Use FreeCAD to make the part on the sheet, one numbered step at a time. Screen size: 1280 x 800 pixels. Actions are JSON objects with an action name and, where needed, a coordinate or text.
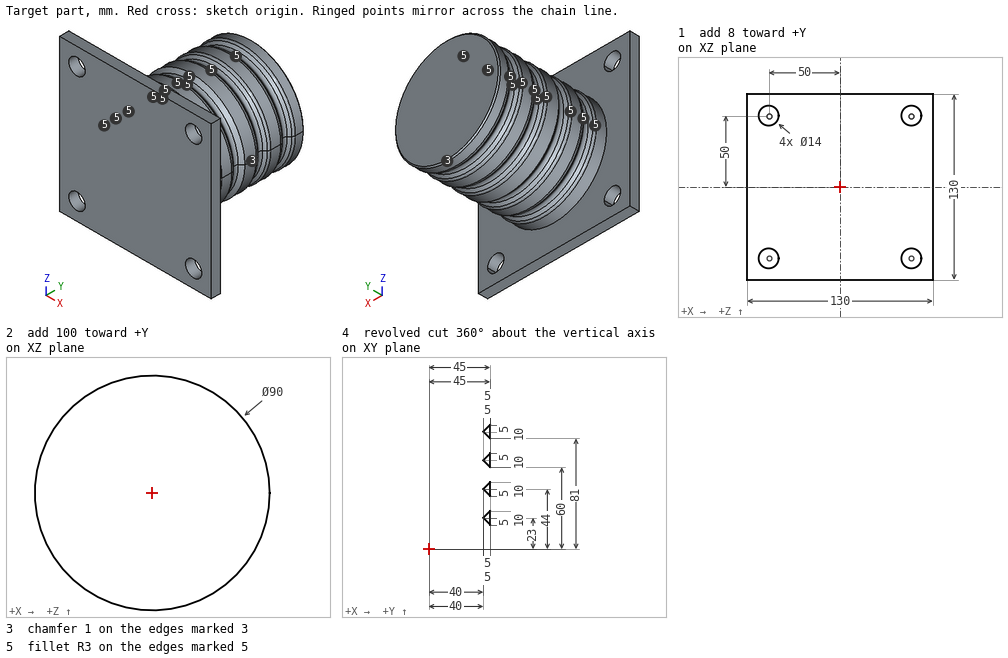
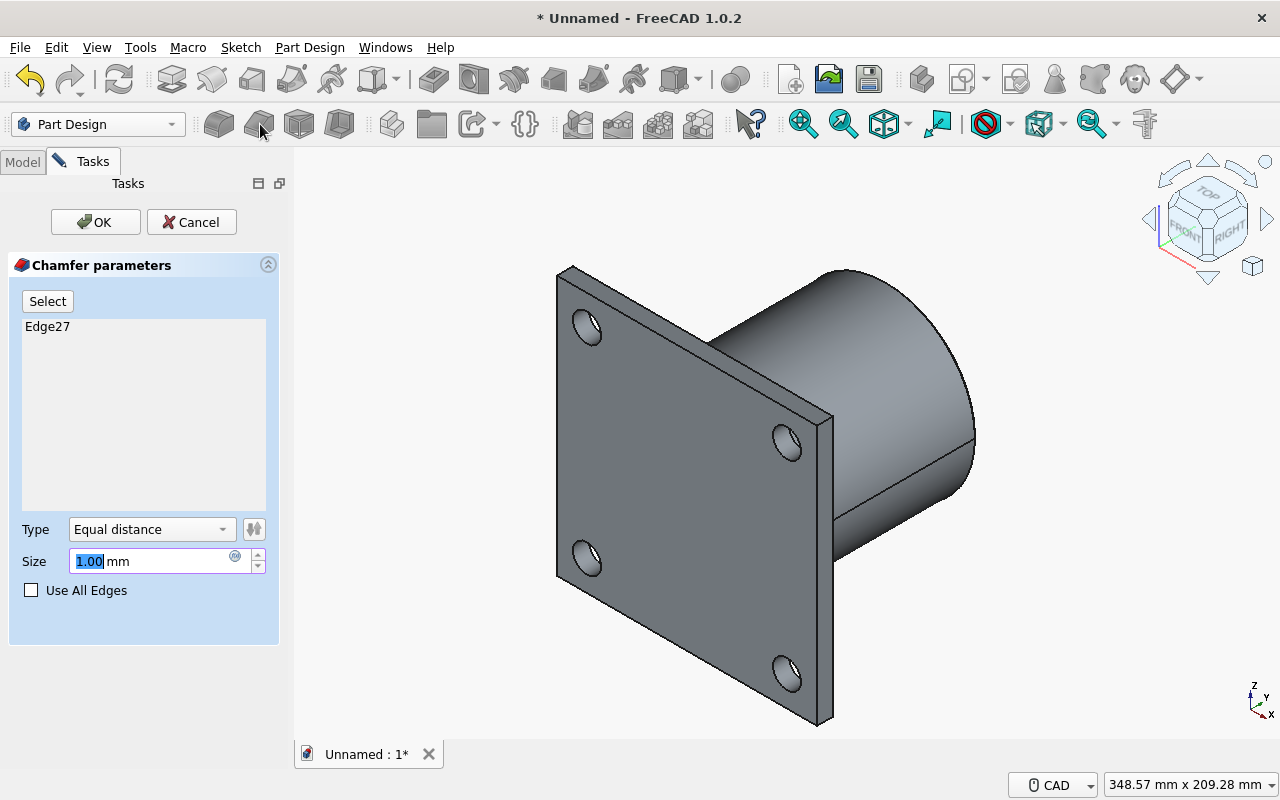
{"action": "type", "text": "1"}
{"action": "key", "text": "Tab"}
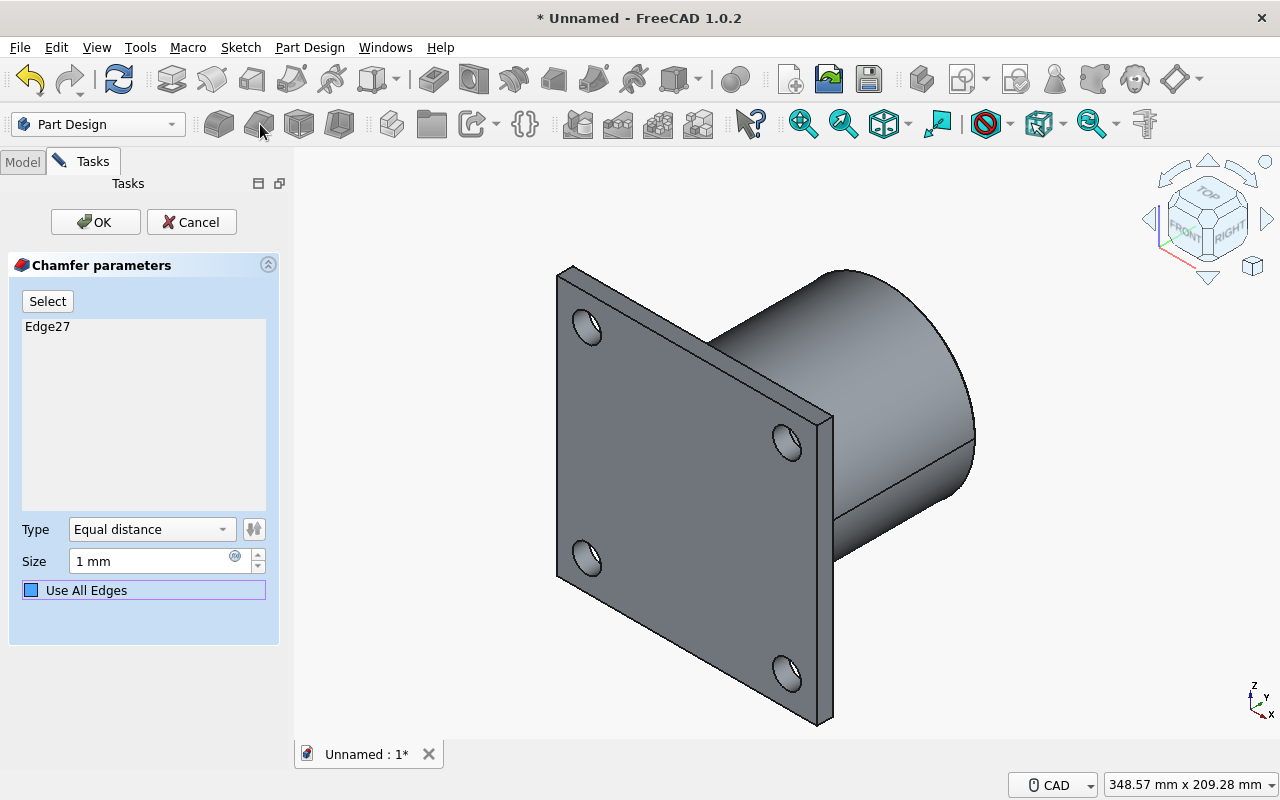
{"action": "left_click", "coordinate": [96, 222]}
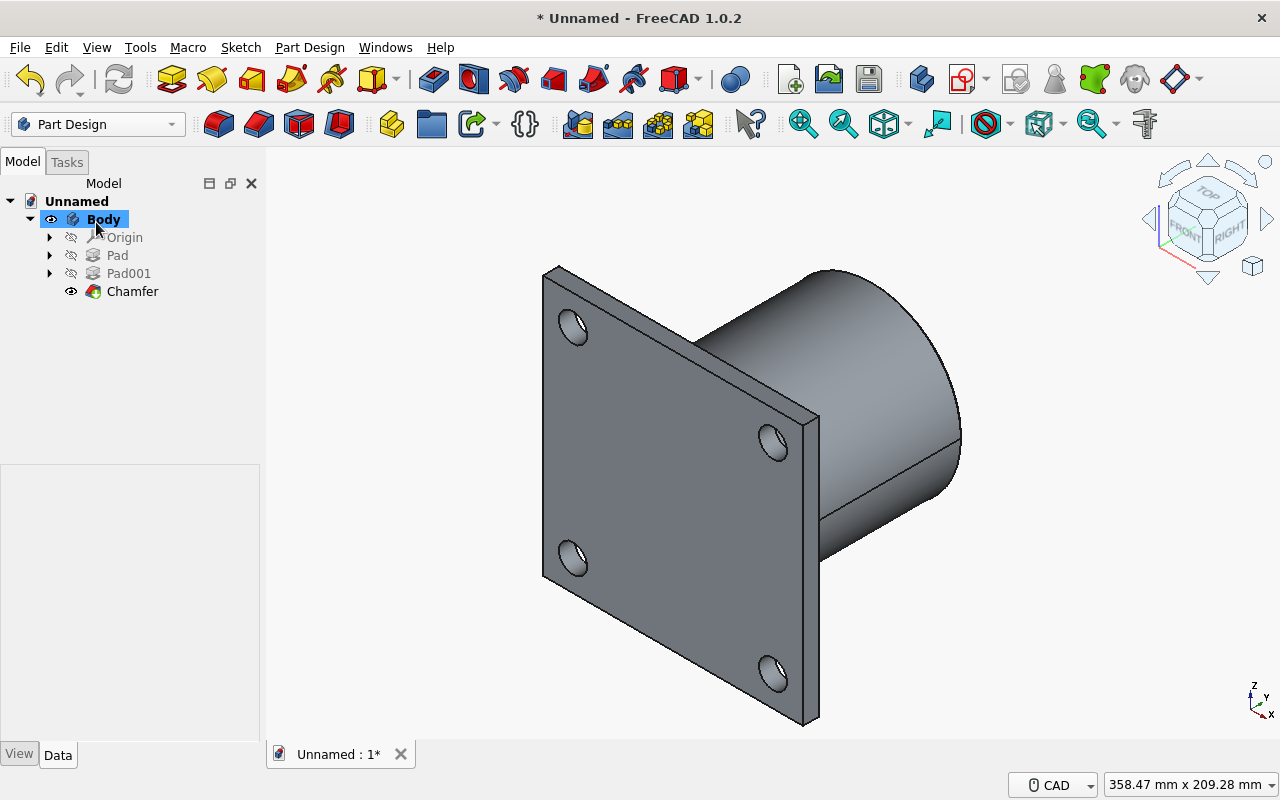
{"action": "left_click", "coordinate": [962, 80]}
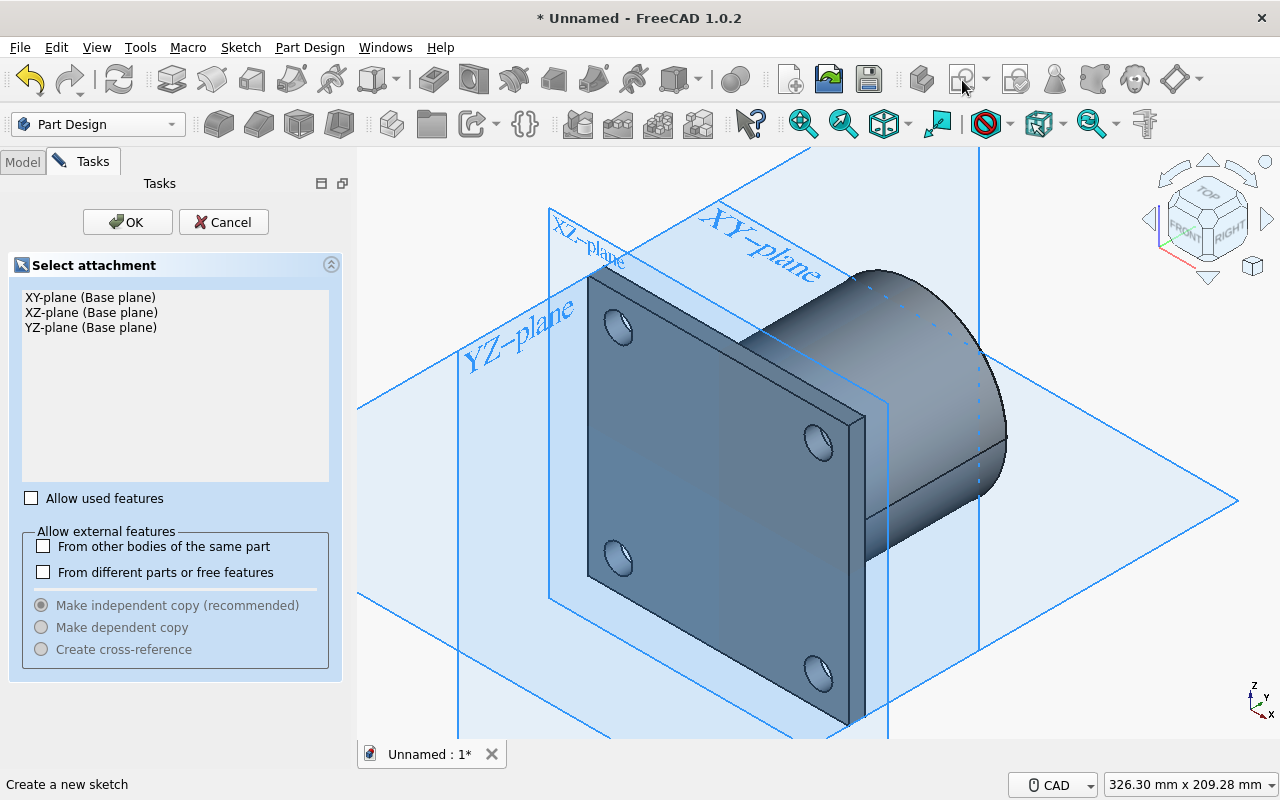
{"action": "left_click", "coordinate": [82, 298]}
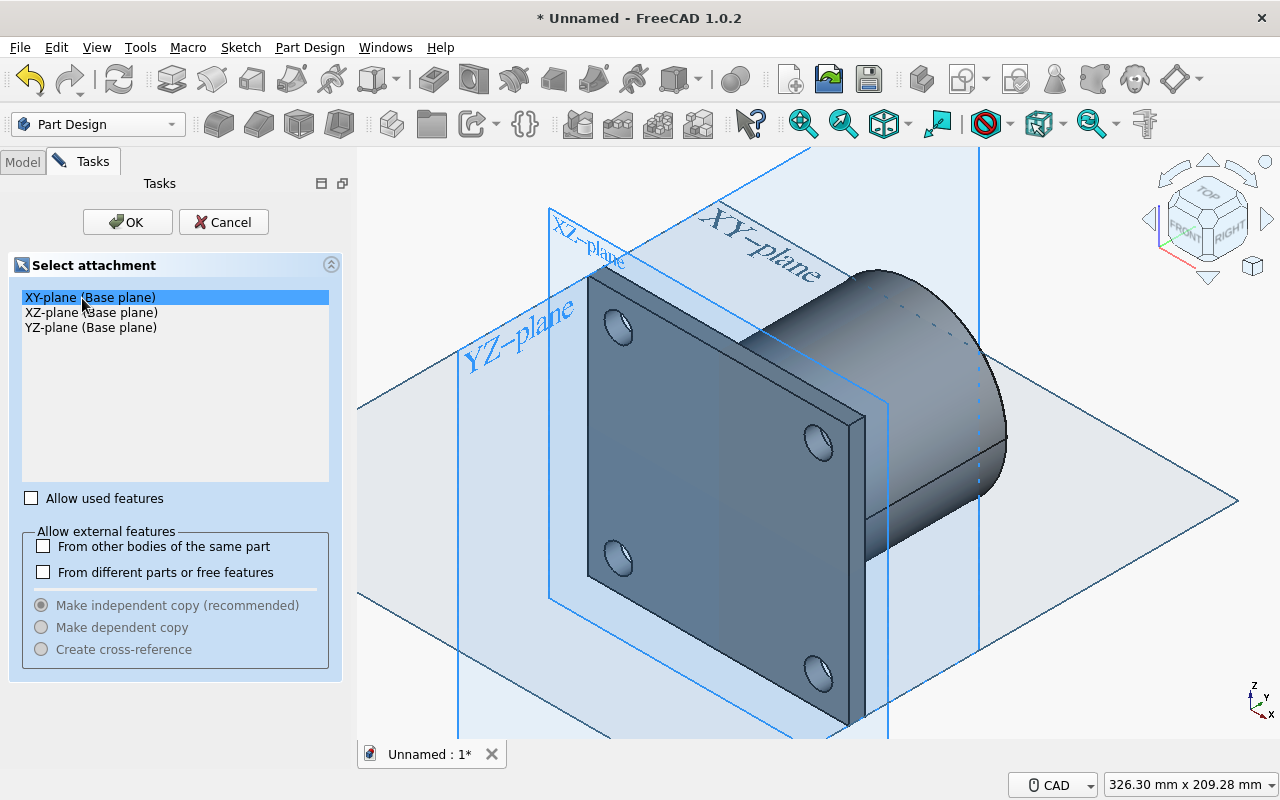
{"action": "left_click", "coordinate": [128, 222]}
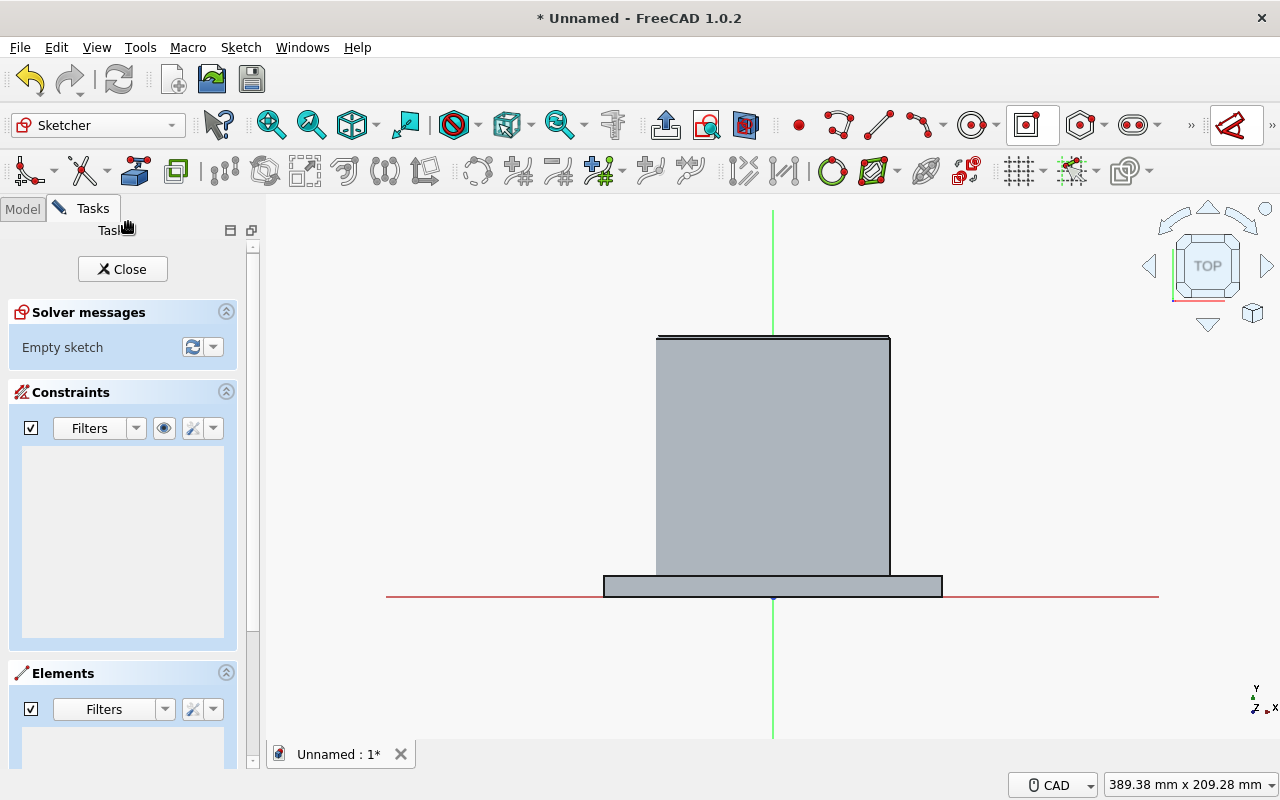
{"action": "left_click", "coordinate": [746, 126]}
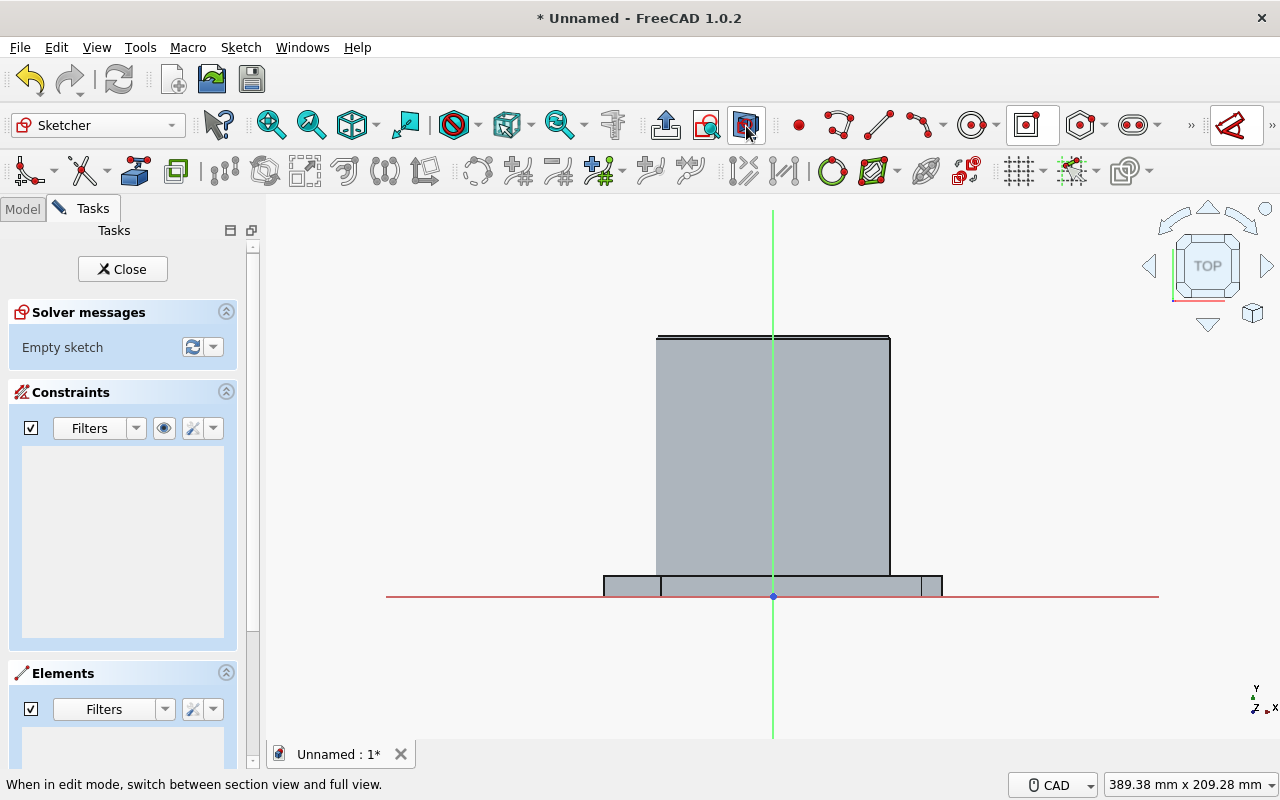
{"action": "scroll", "coordinate": [1090, 502], "scroll_direction": "up", "scroll_amount": 2}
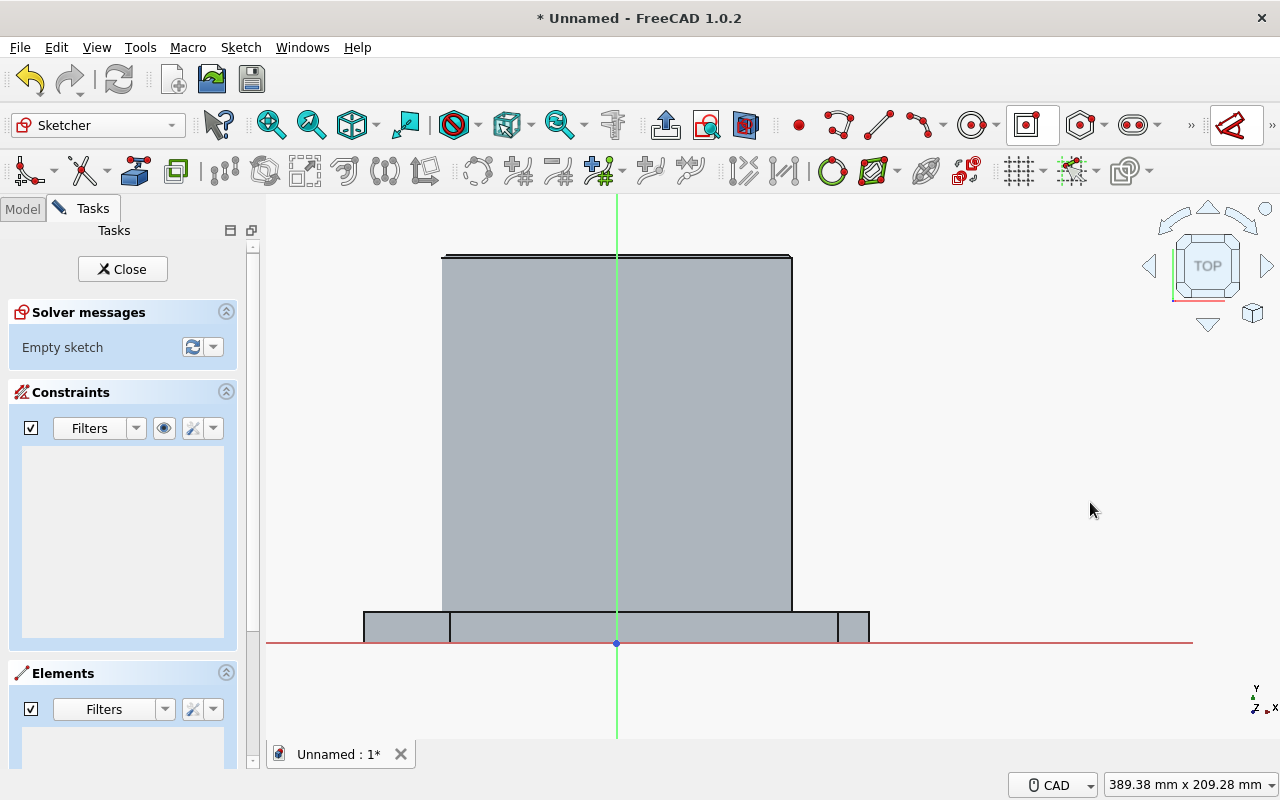
{"action": "left_click", "coordinate": [840, 126]}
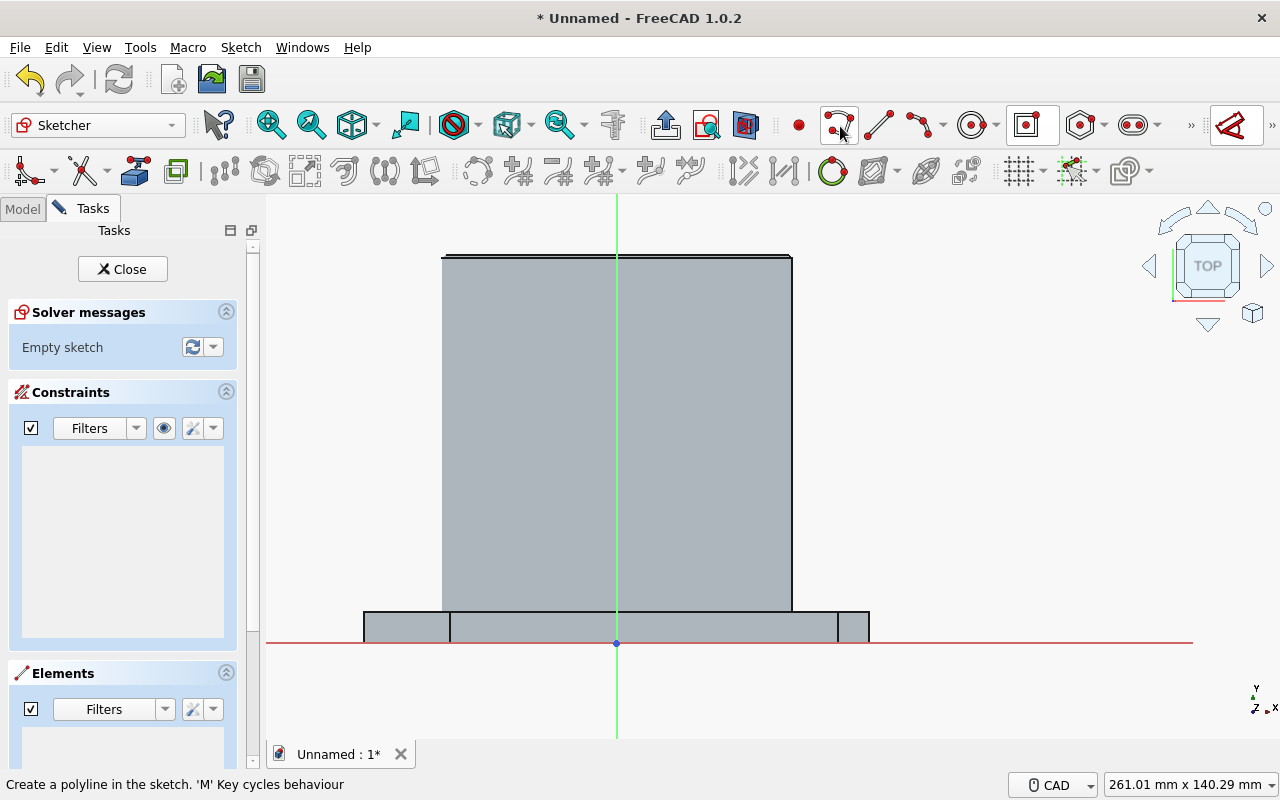
{"action": "left_click", "coordinate": [772, 554]}
{"action": "left_click", "coordinate": [792, 573]}
{"action": "left_click", "coordinate": [792, 534]}
{"action": "left_click", "coordinate": [772, 555]}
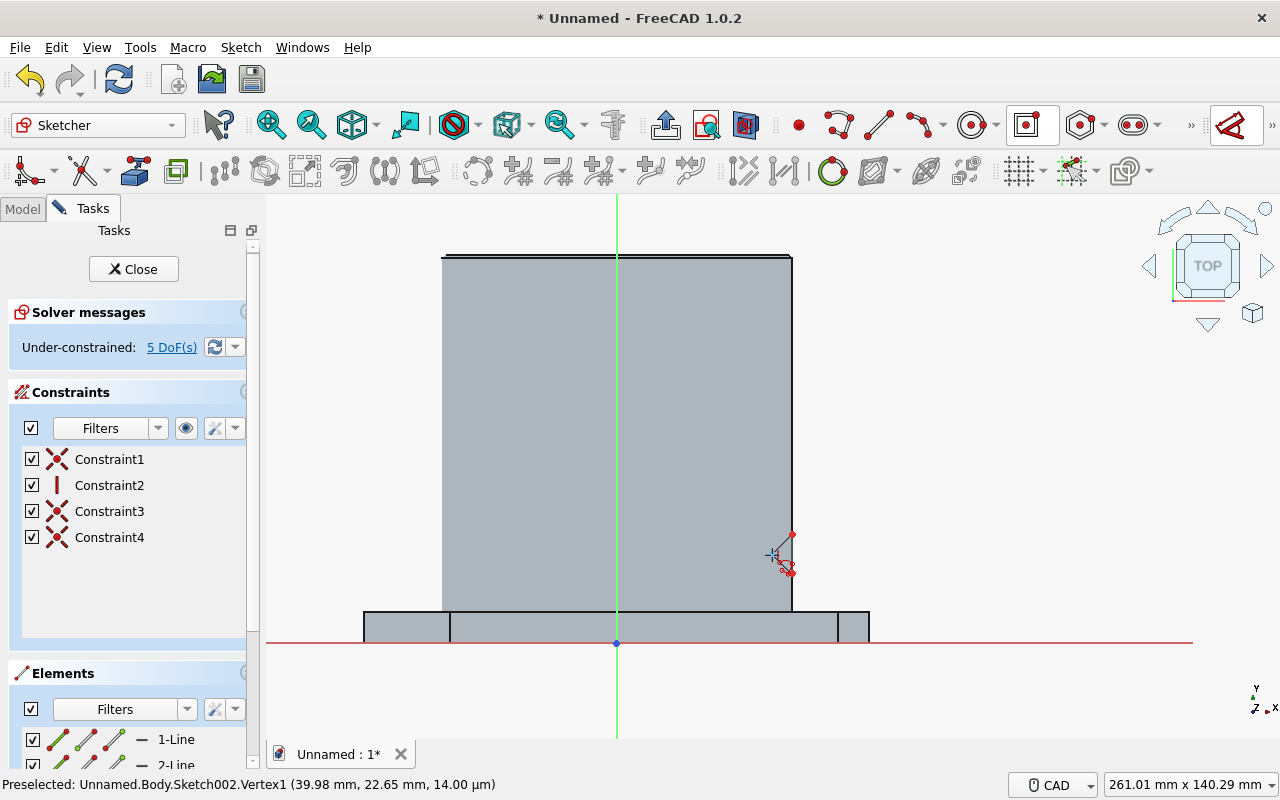
{"action": "left_click", "coordinate": [772, 472]}
{"action": "left_click", "coordinate": [792, 491]}
{"action": "left_click", "coordinate": [792, 453]}
{"action": "left_click", "coordinate": [772, 473]}